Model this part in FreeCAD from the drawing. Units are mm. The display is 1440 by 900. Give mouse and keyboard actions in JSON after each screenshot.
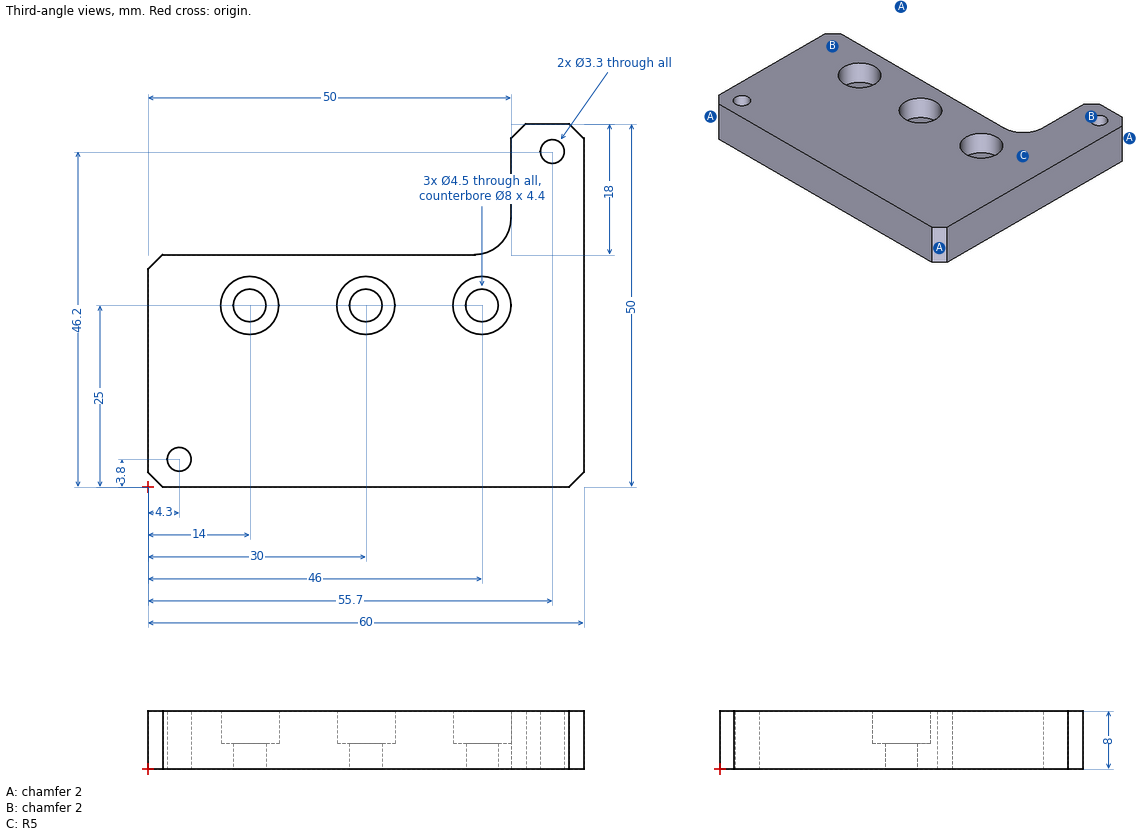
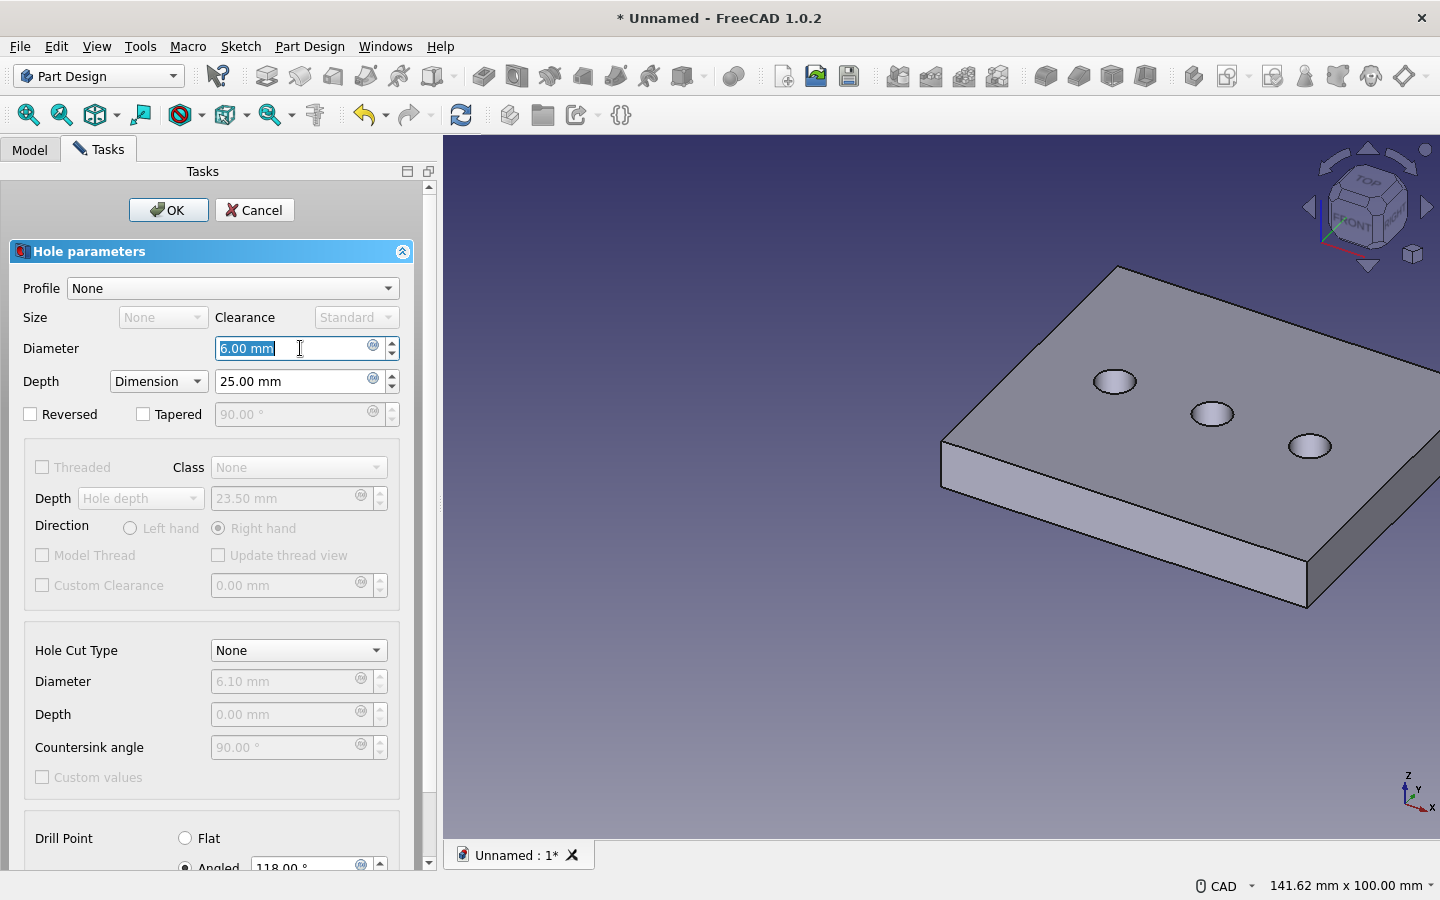
{"action": "type", "text": "4.5"}
{"action": "key", "text": "Tab"}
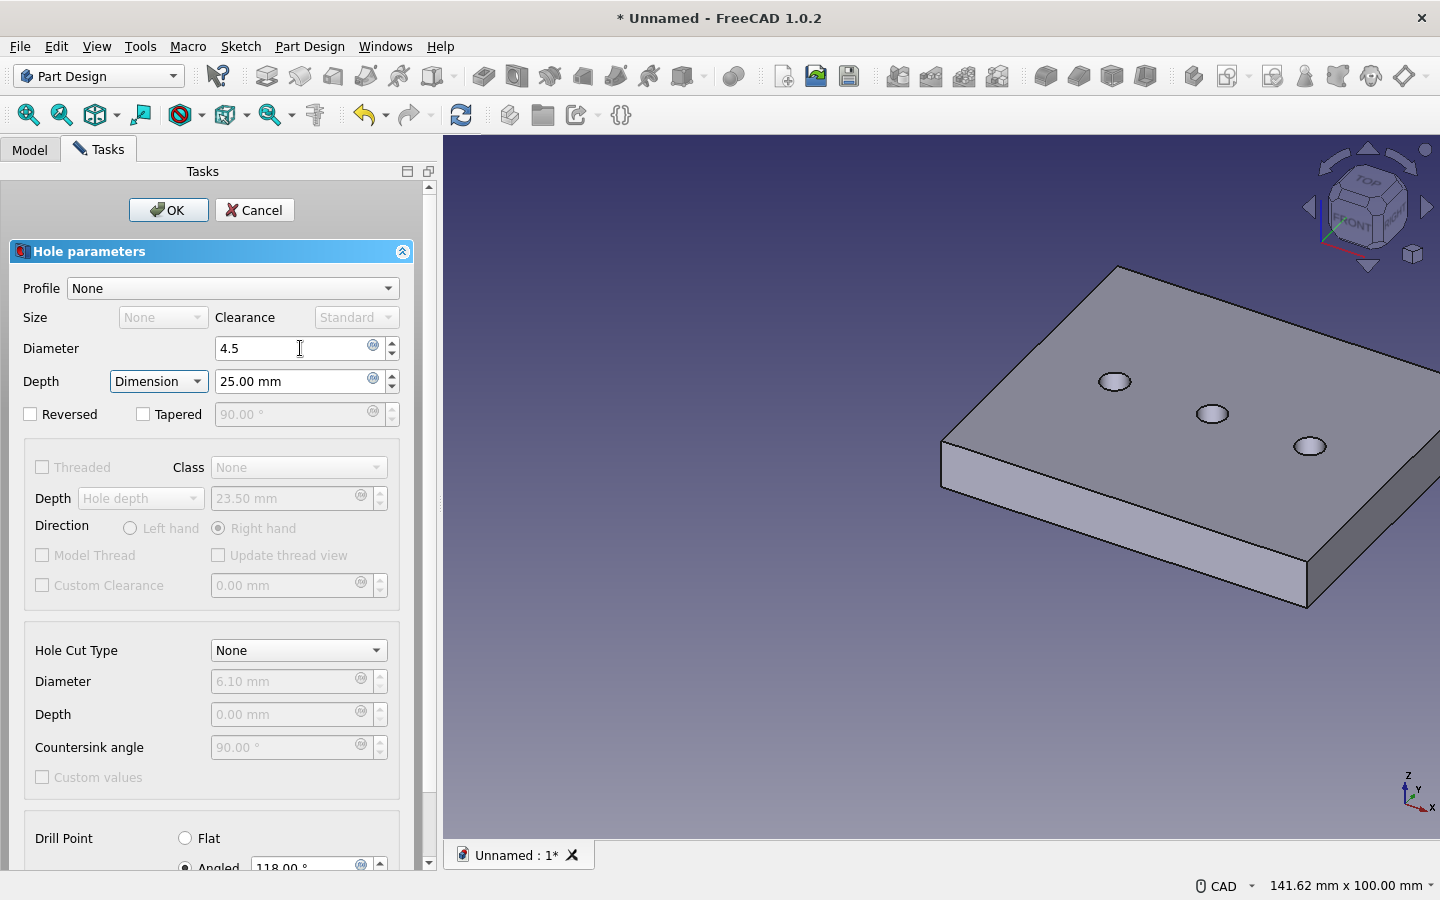
{"action": "left_click", "coordinate": [160, 382]}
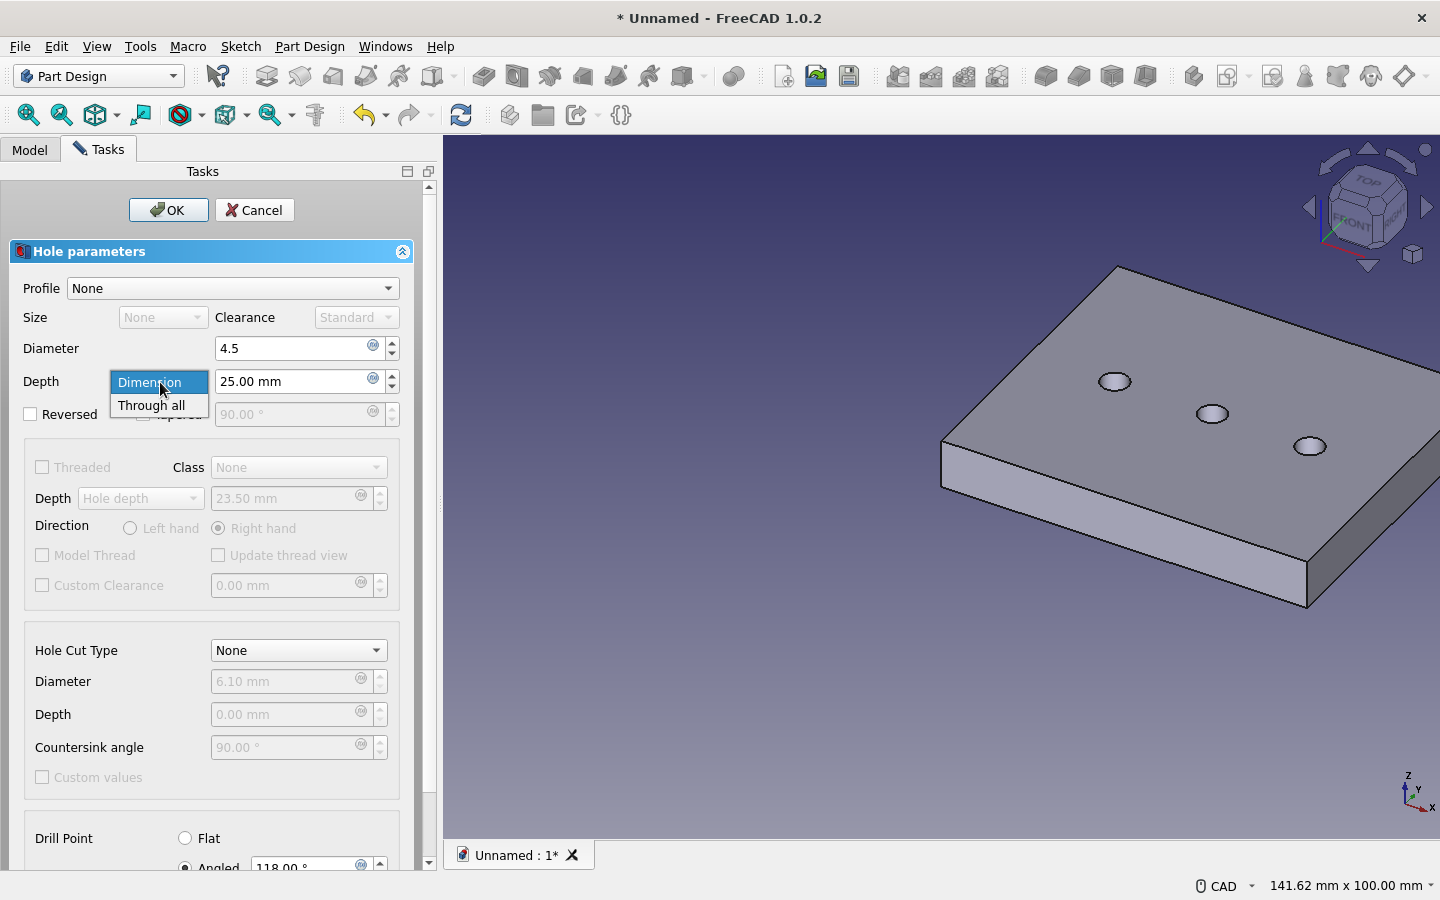
{"action": "left_click", "coordinate": [158, 406]}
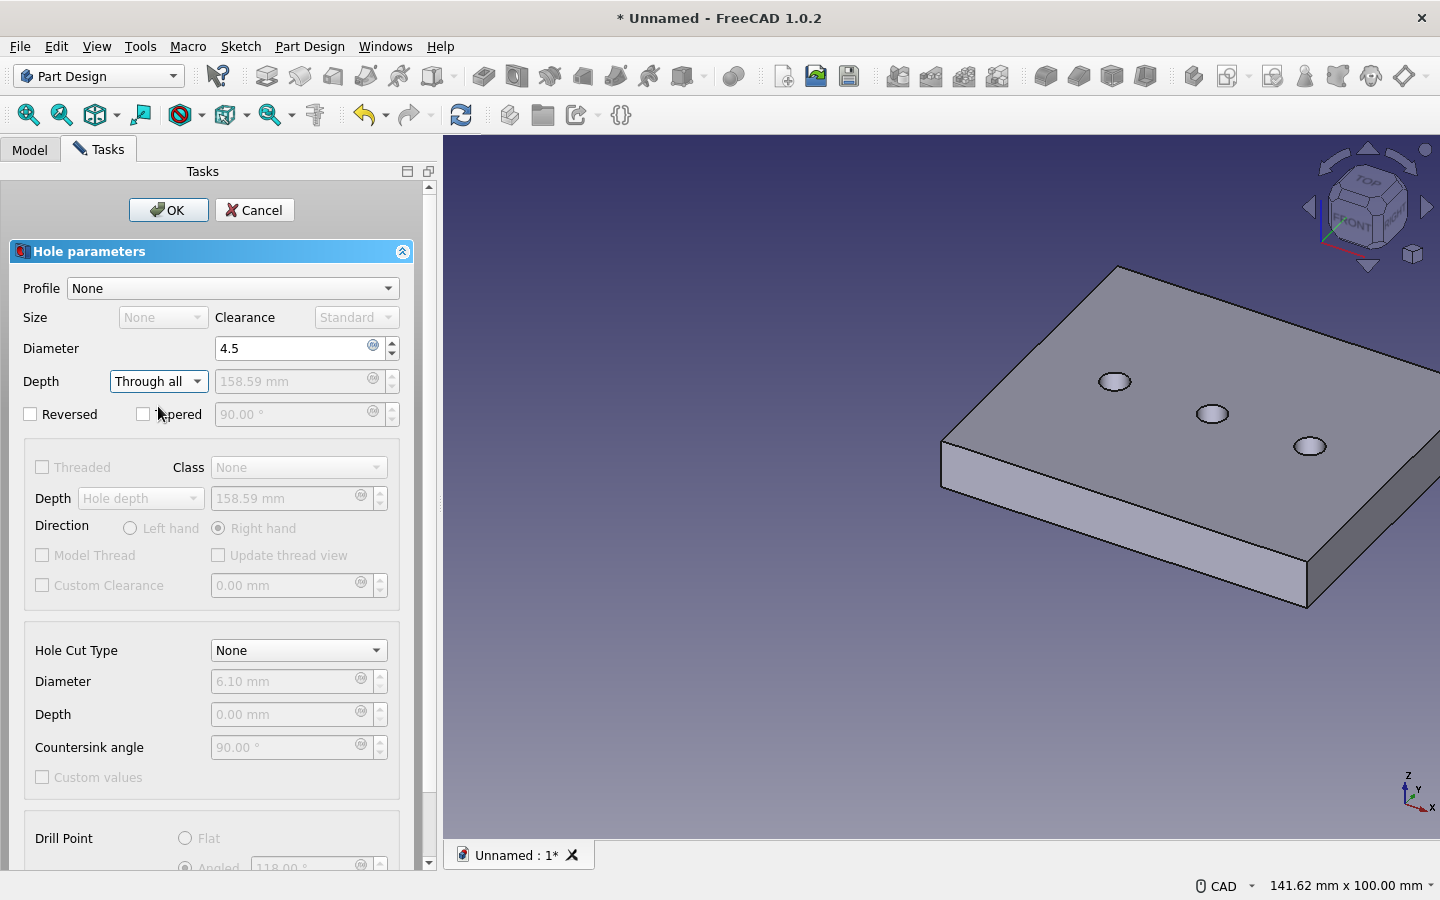
{"action": "left_click", "coordinate": [300, 650]}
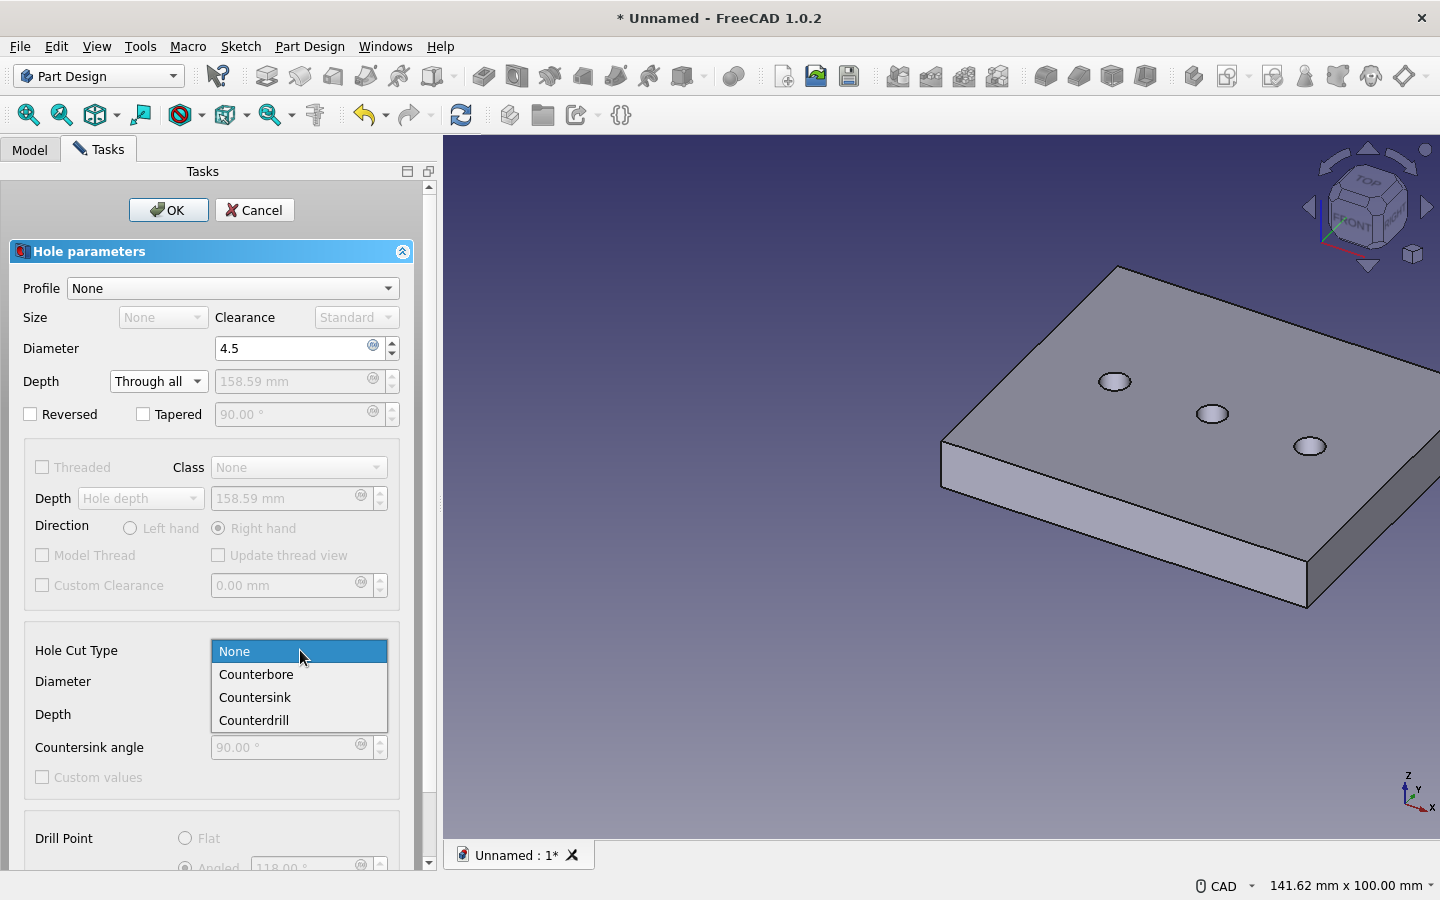
{"action": "left_click", "coordinate": [298, 674]}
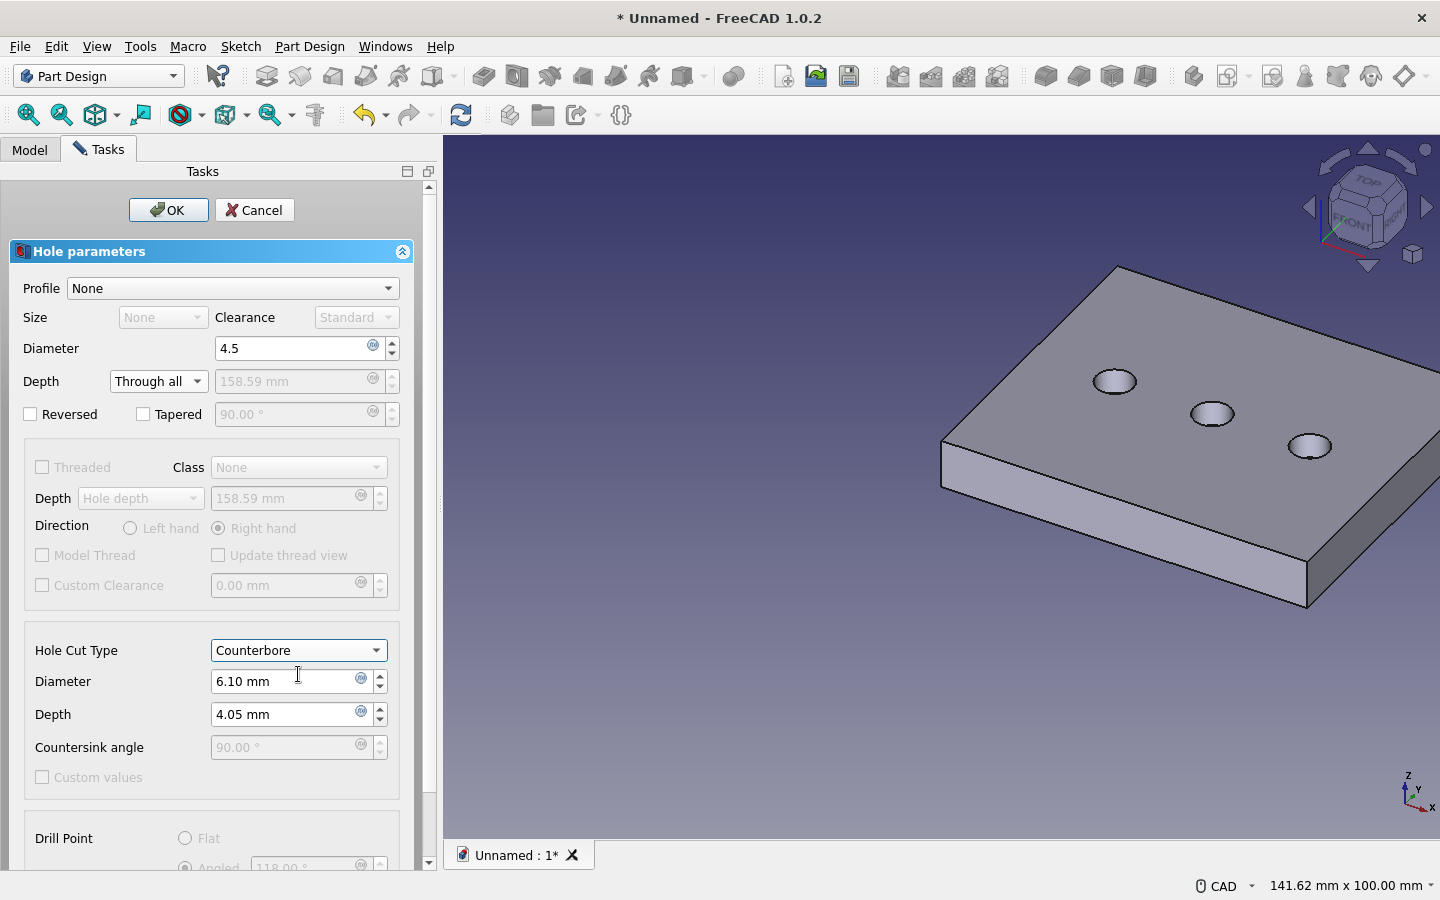
{"action": "triple_click", "coordinate": [292, 682]}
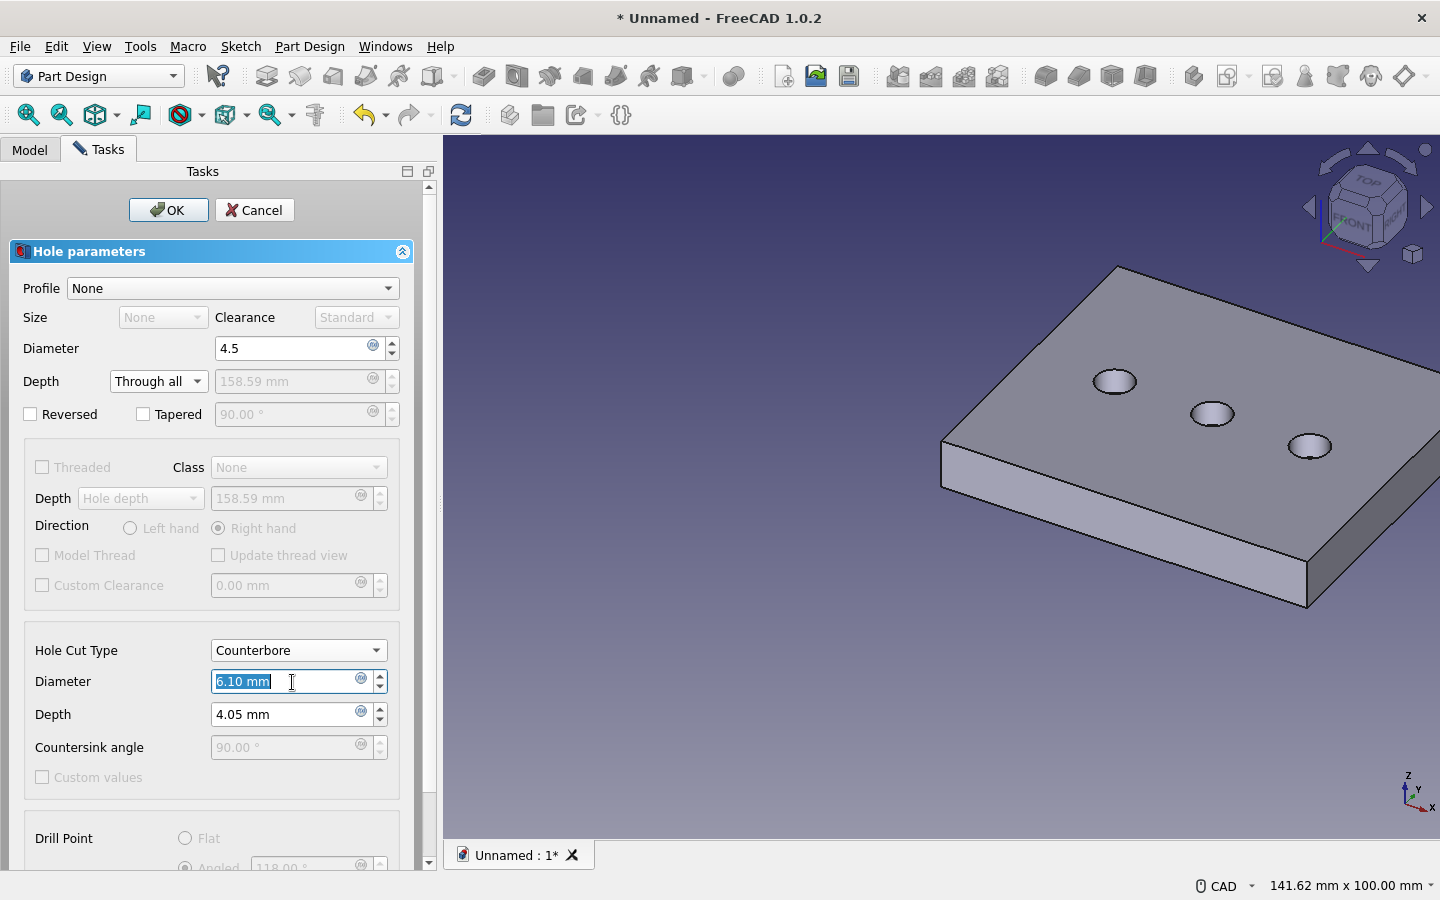
{"action": "type", "text": "8"}
{"action": "key", "text": "Tab"}